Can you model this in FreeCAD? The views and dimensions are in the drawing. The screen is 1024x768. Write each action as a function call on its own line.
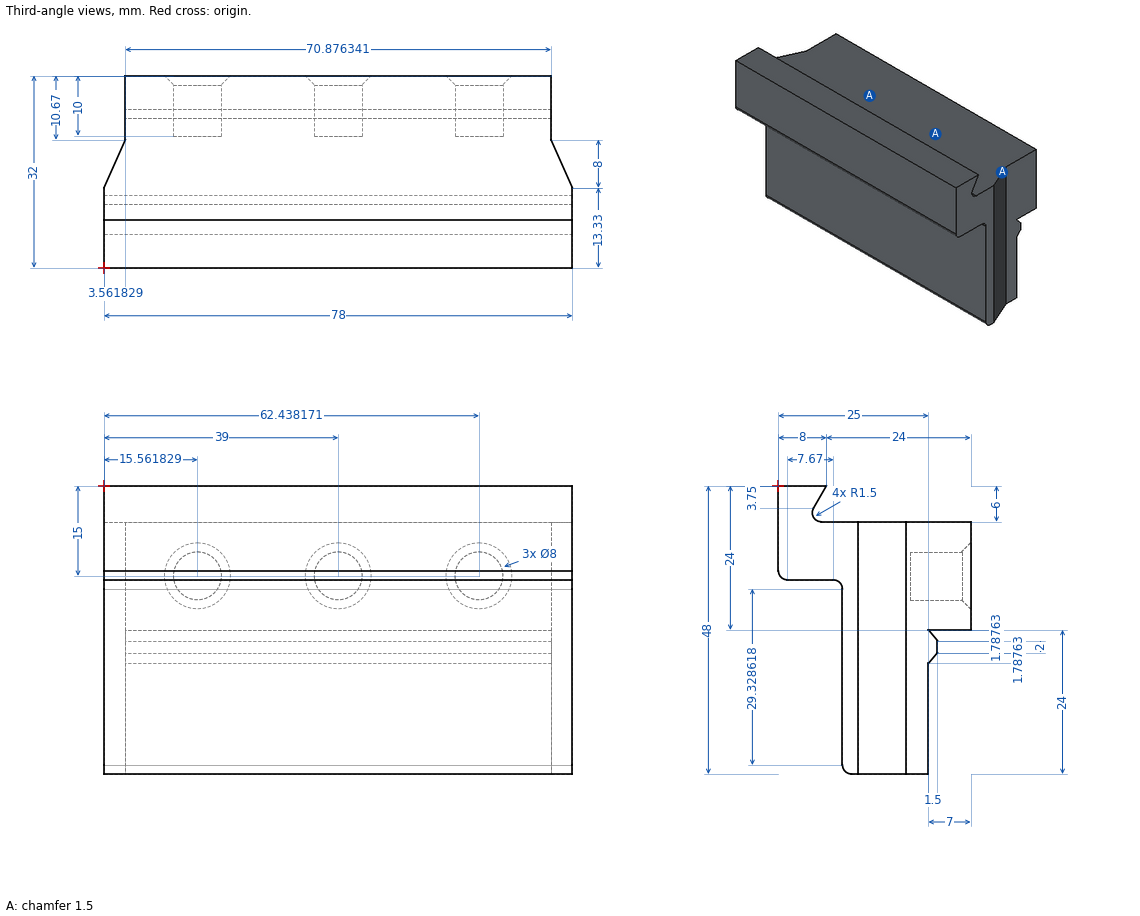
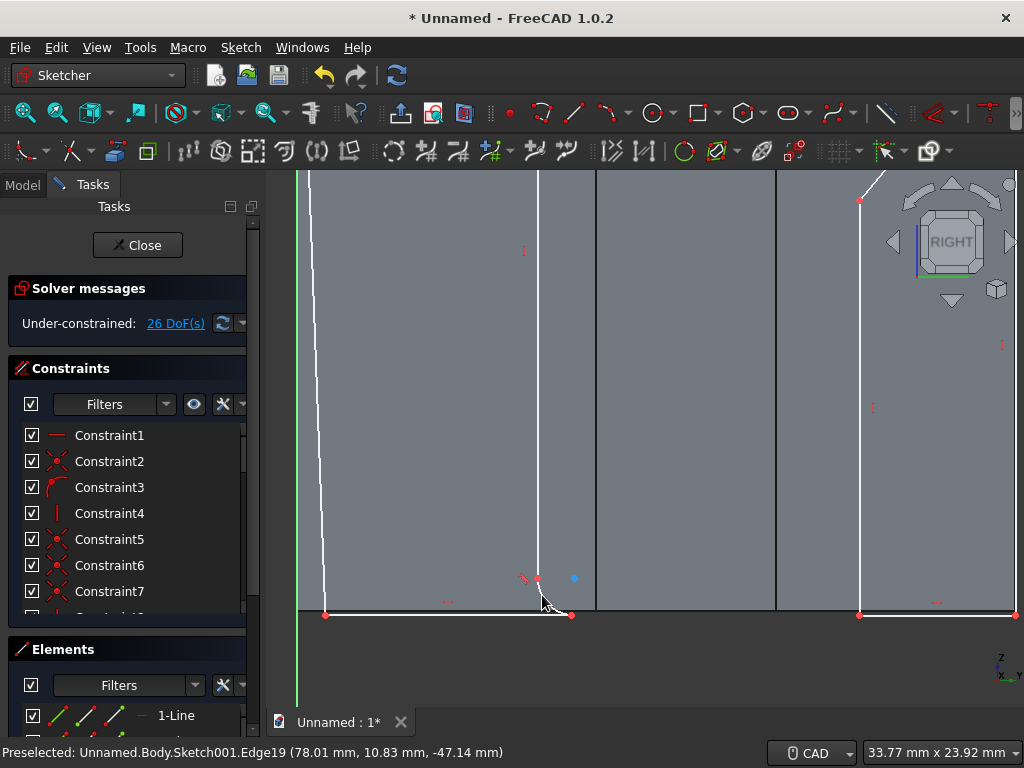
scroll(542, 596, down, 6)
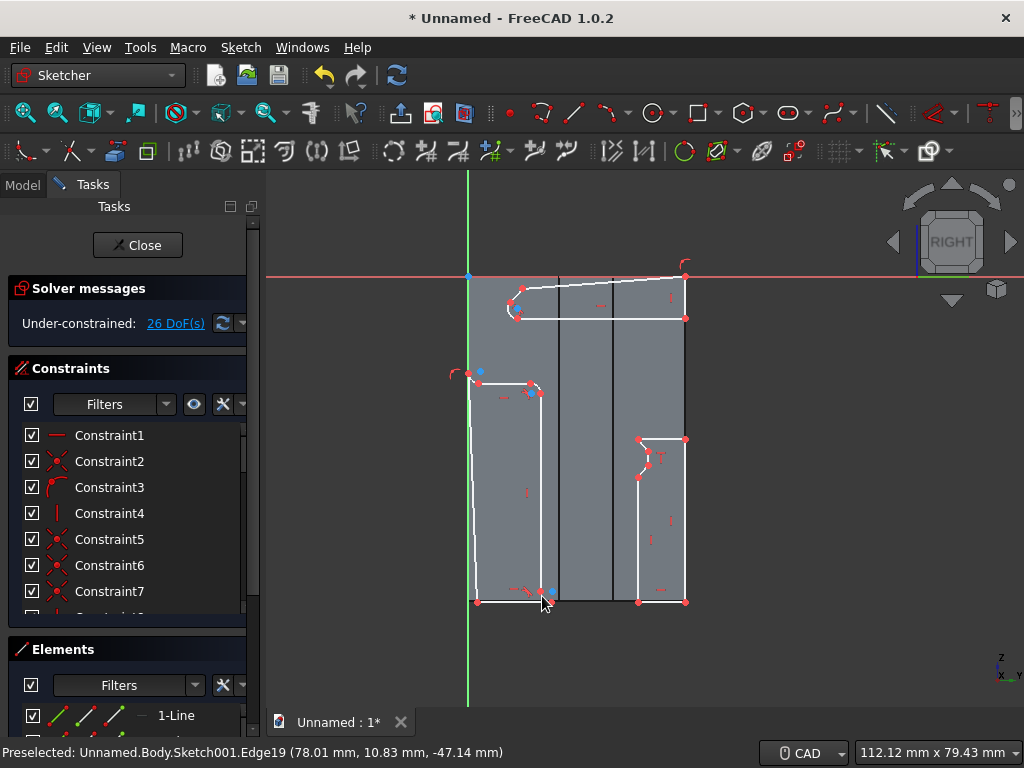
click(515, 384)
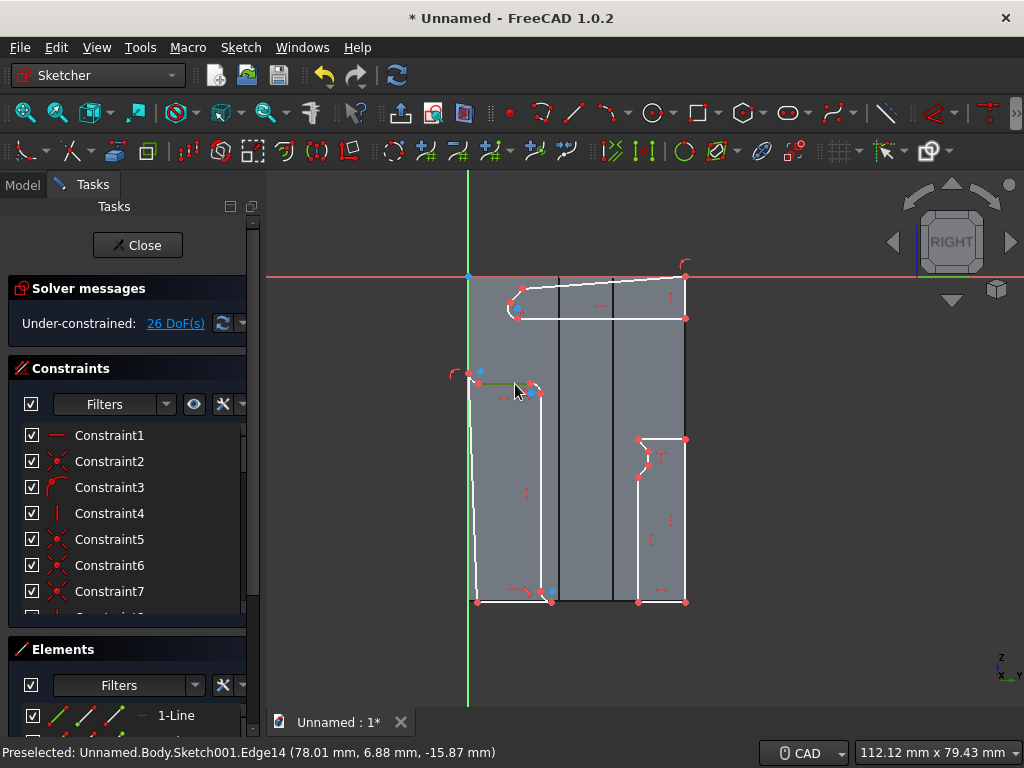
scroll(538, 386, up, 3)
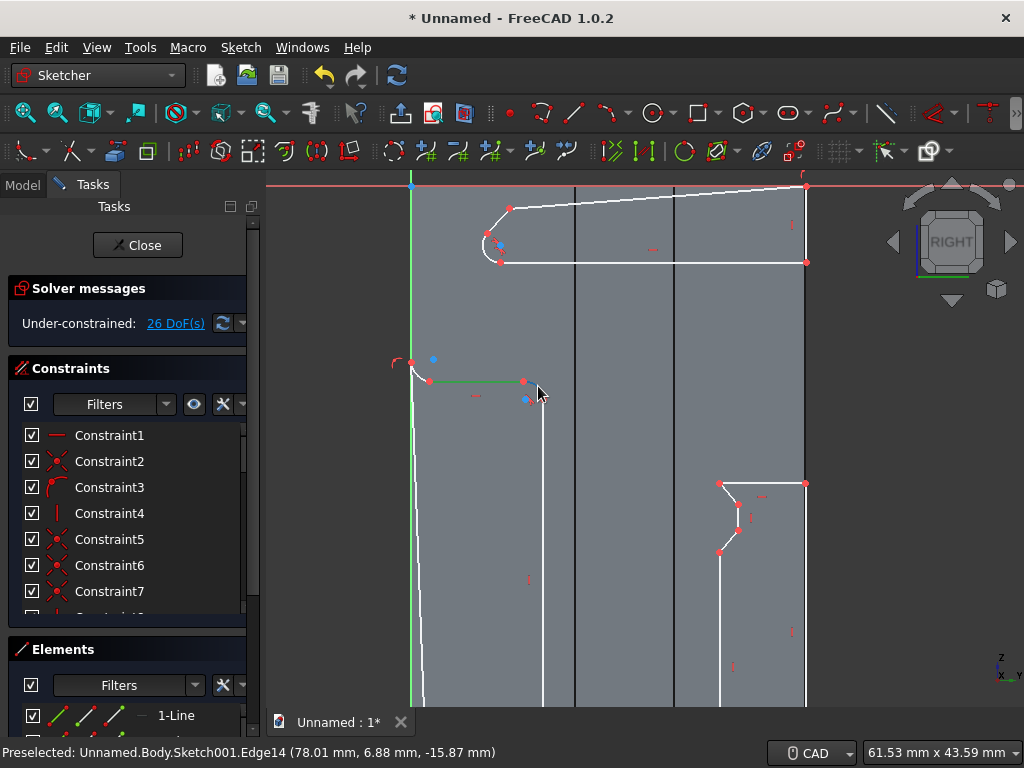
click(537, 386)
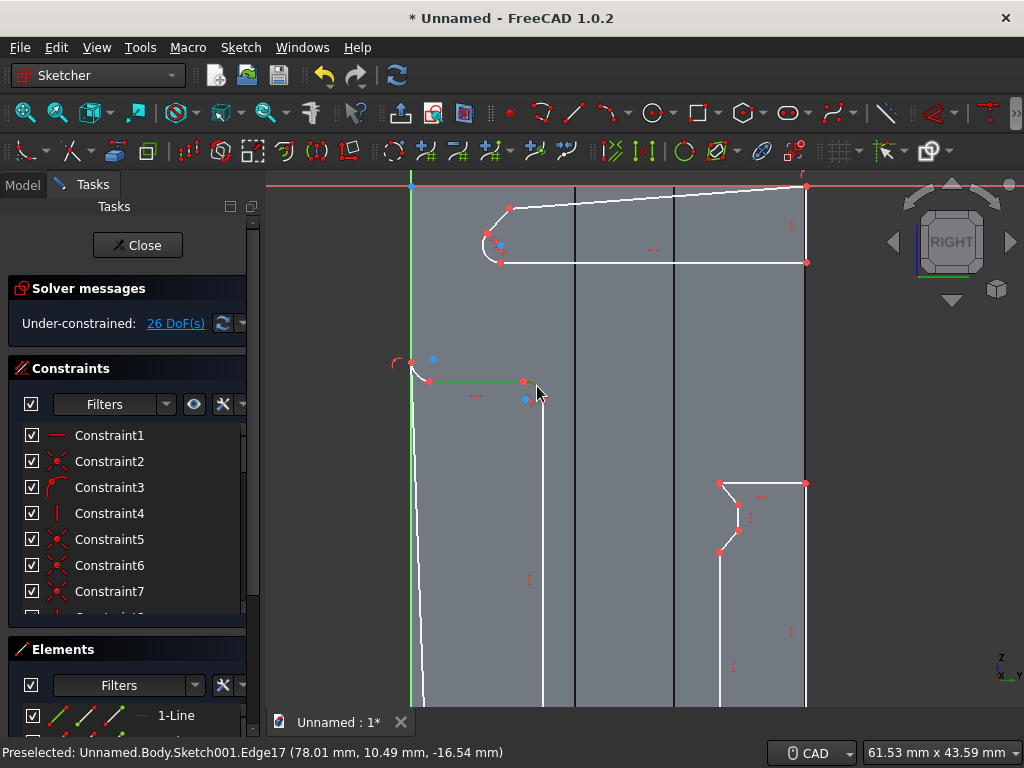
key(t)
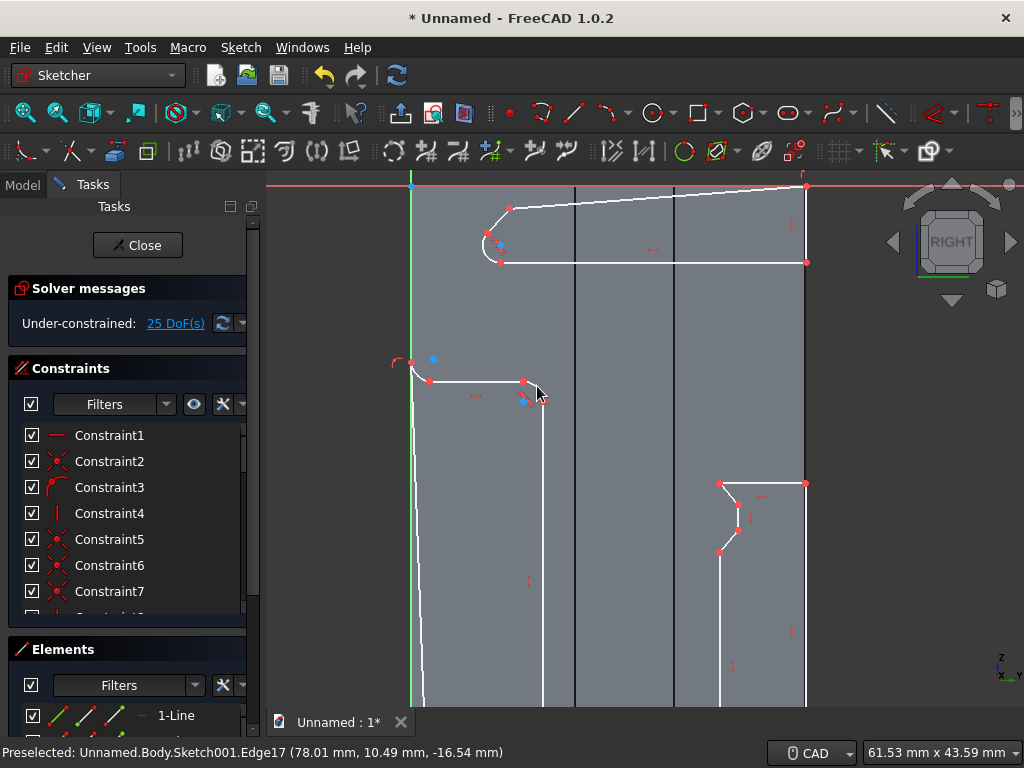
click(495, 382)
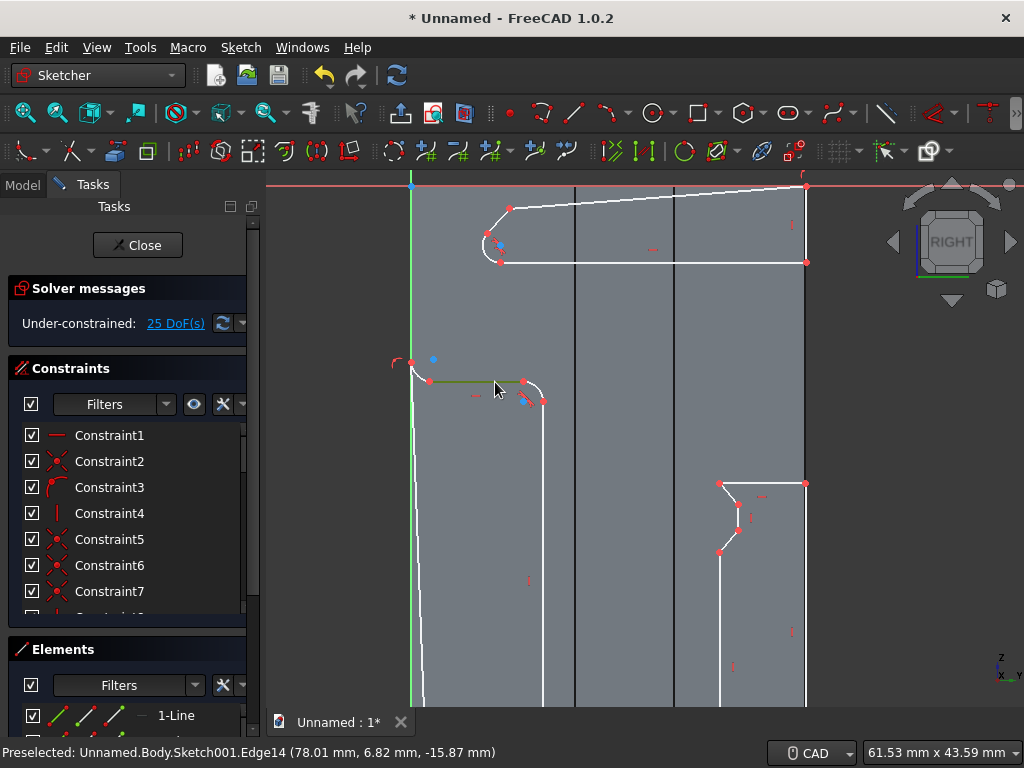
scroll(421, 379, up, 3)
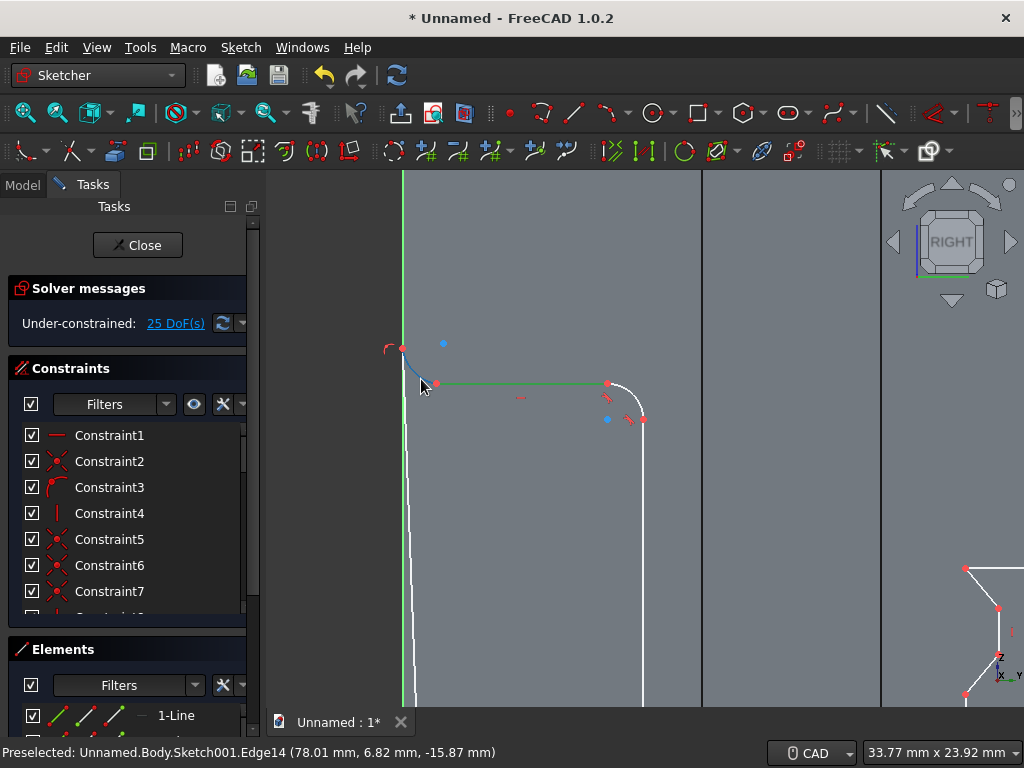
click(422, 378)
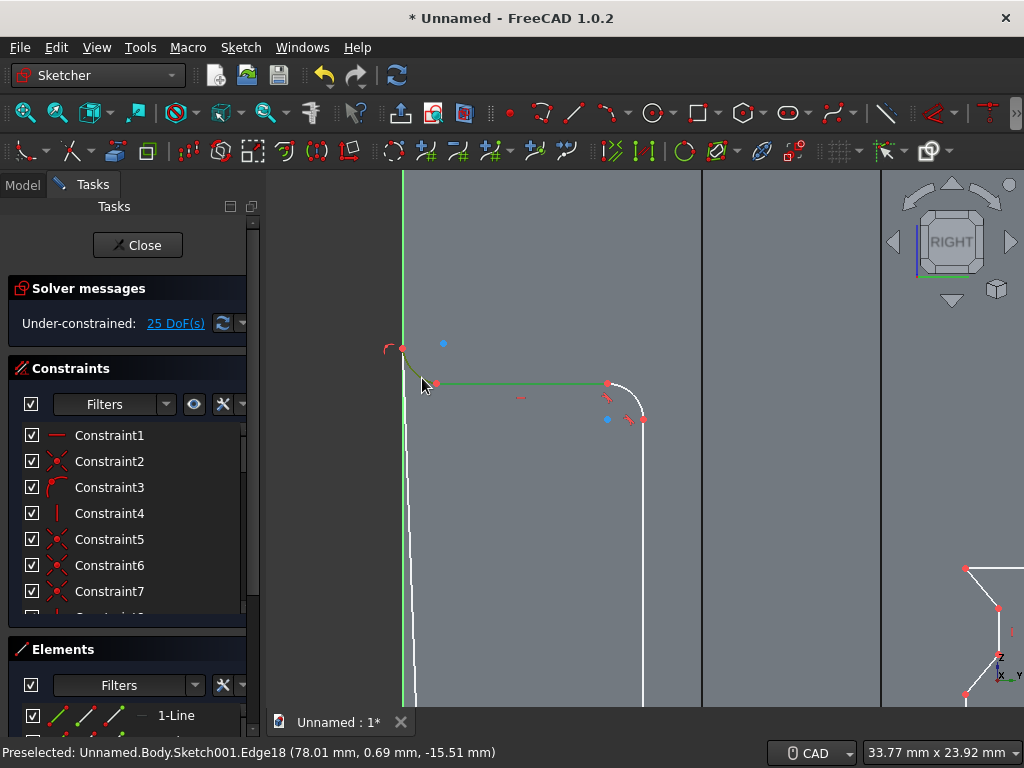
key(t)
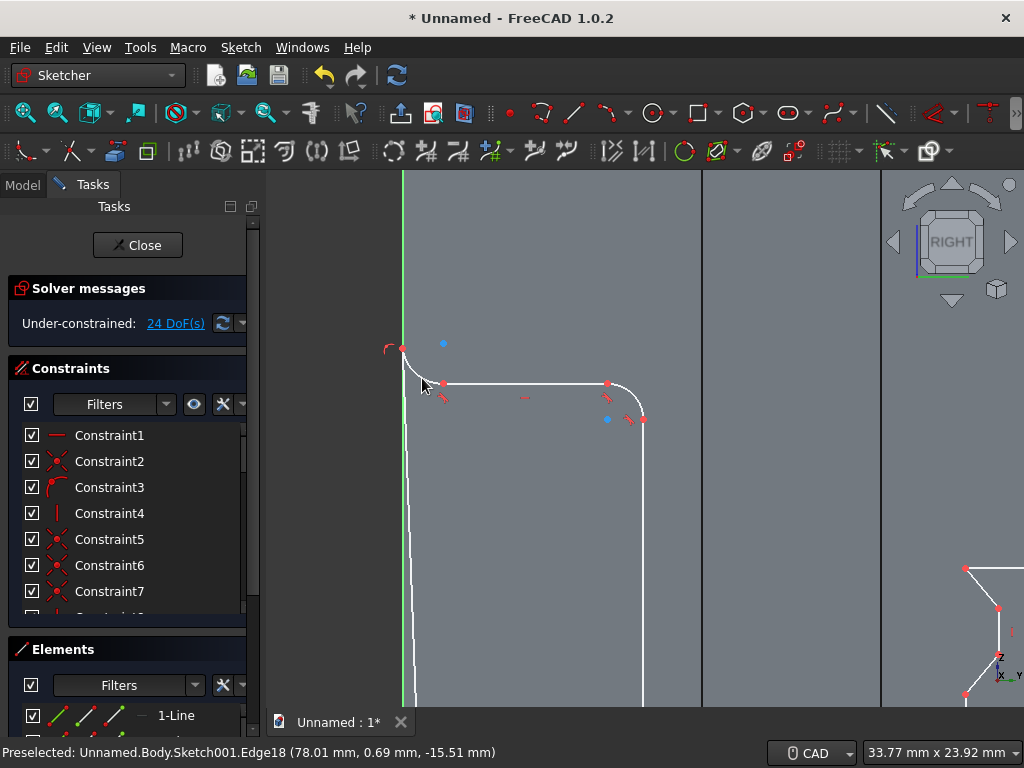
click(414, 653)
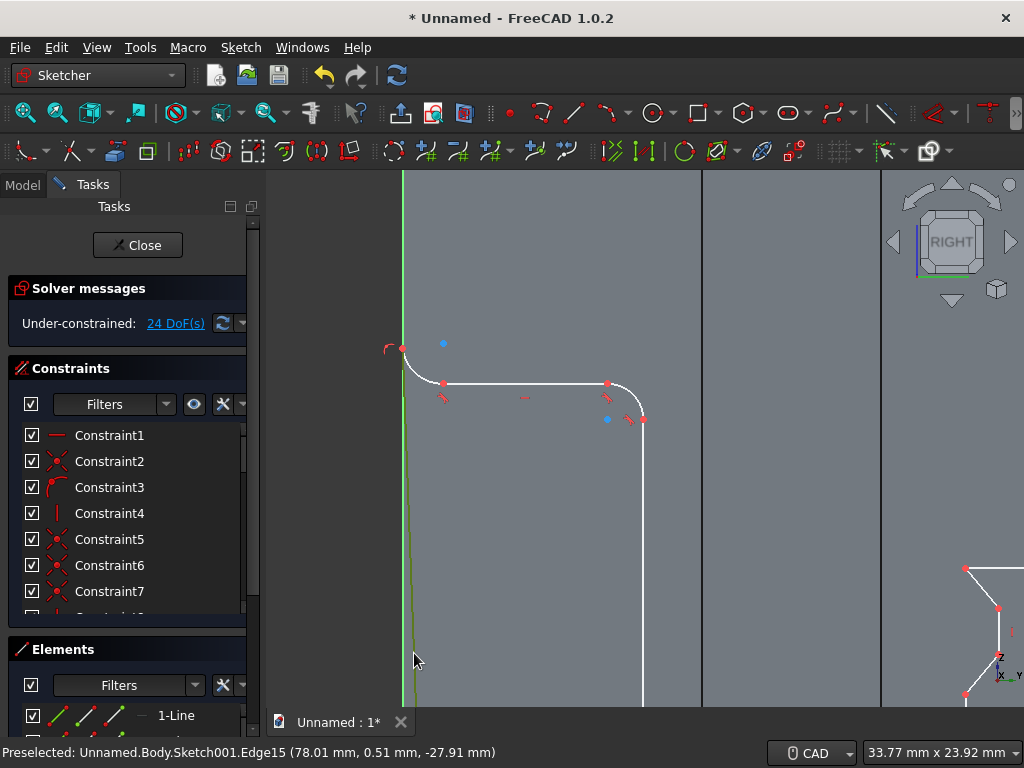
click(426, 380)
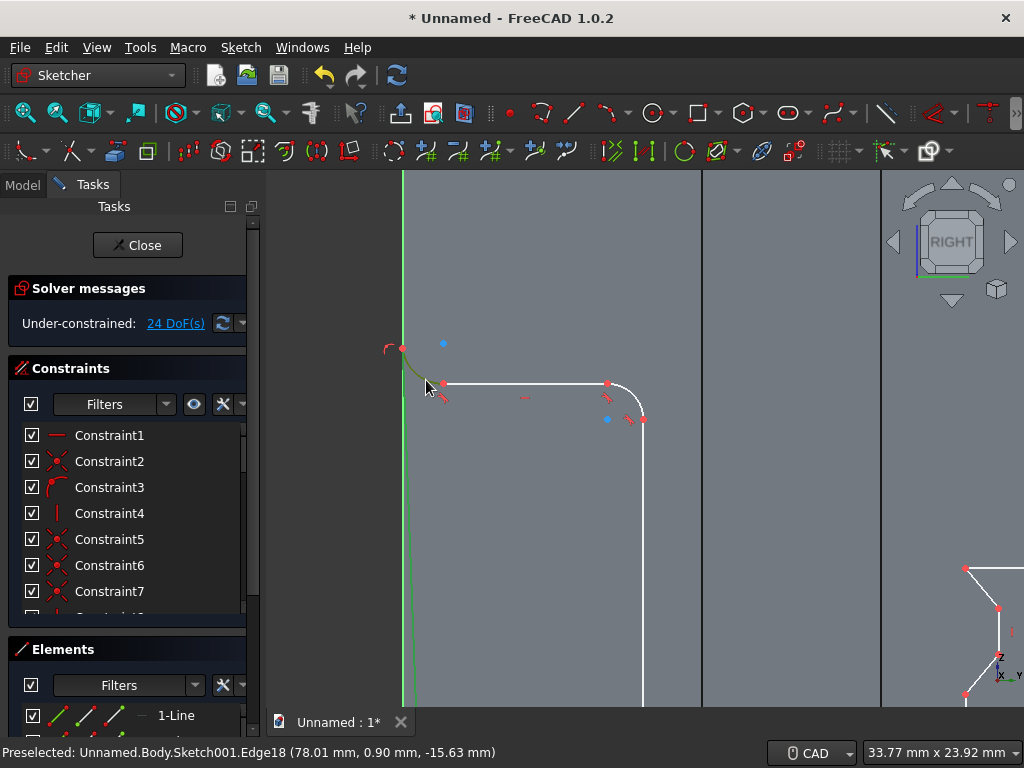
key(t)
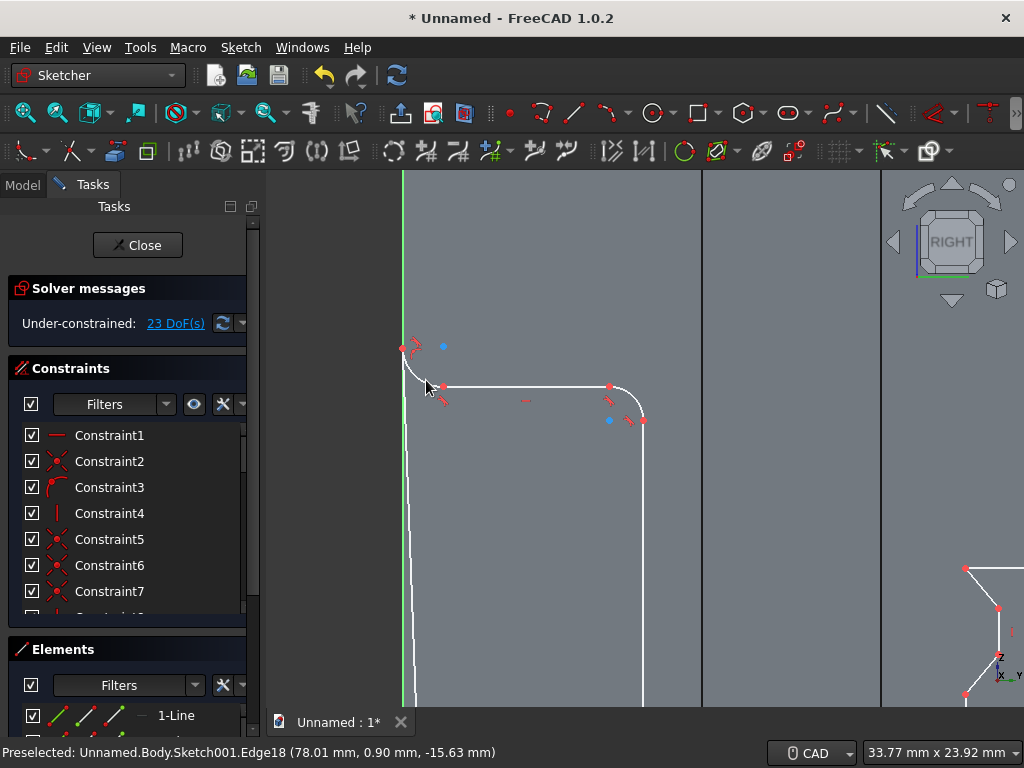
scroll(497, 383, down, 6)